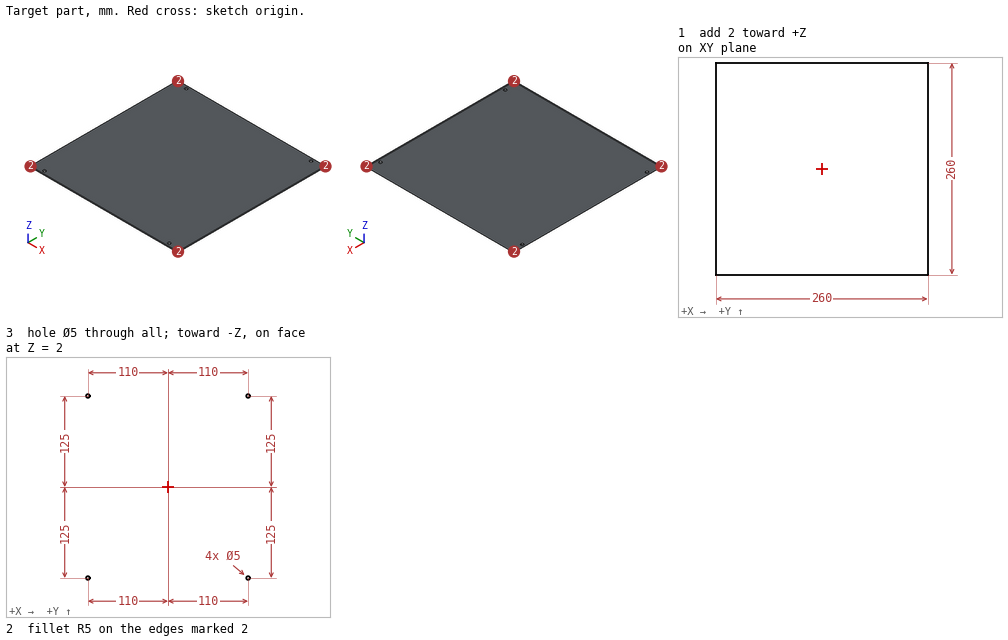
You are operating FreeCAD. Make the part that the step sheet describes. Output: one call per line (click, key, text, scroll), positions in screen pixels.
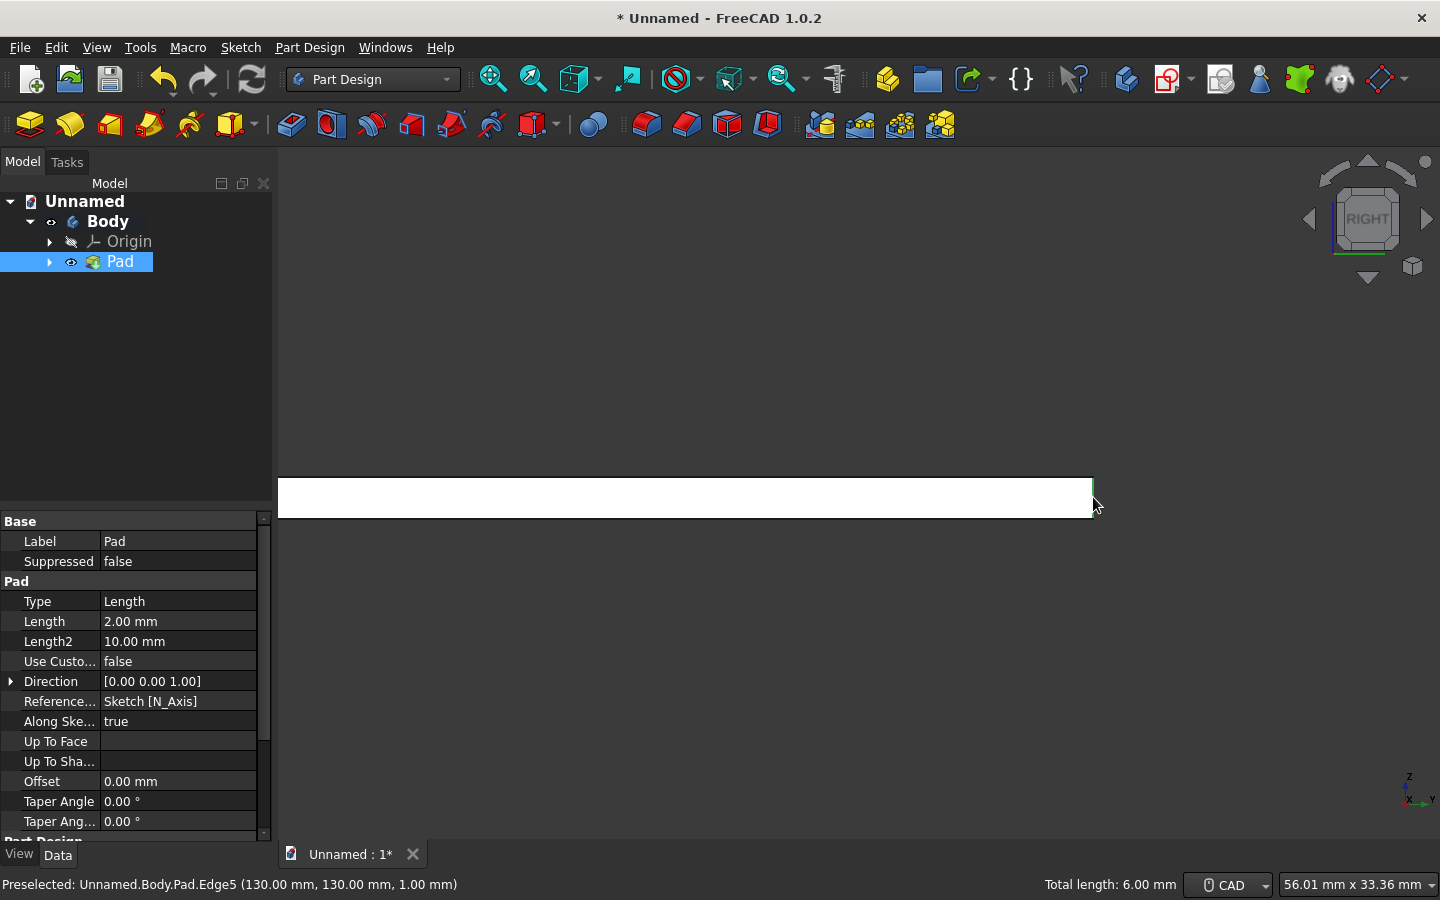
click(494, 80)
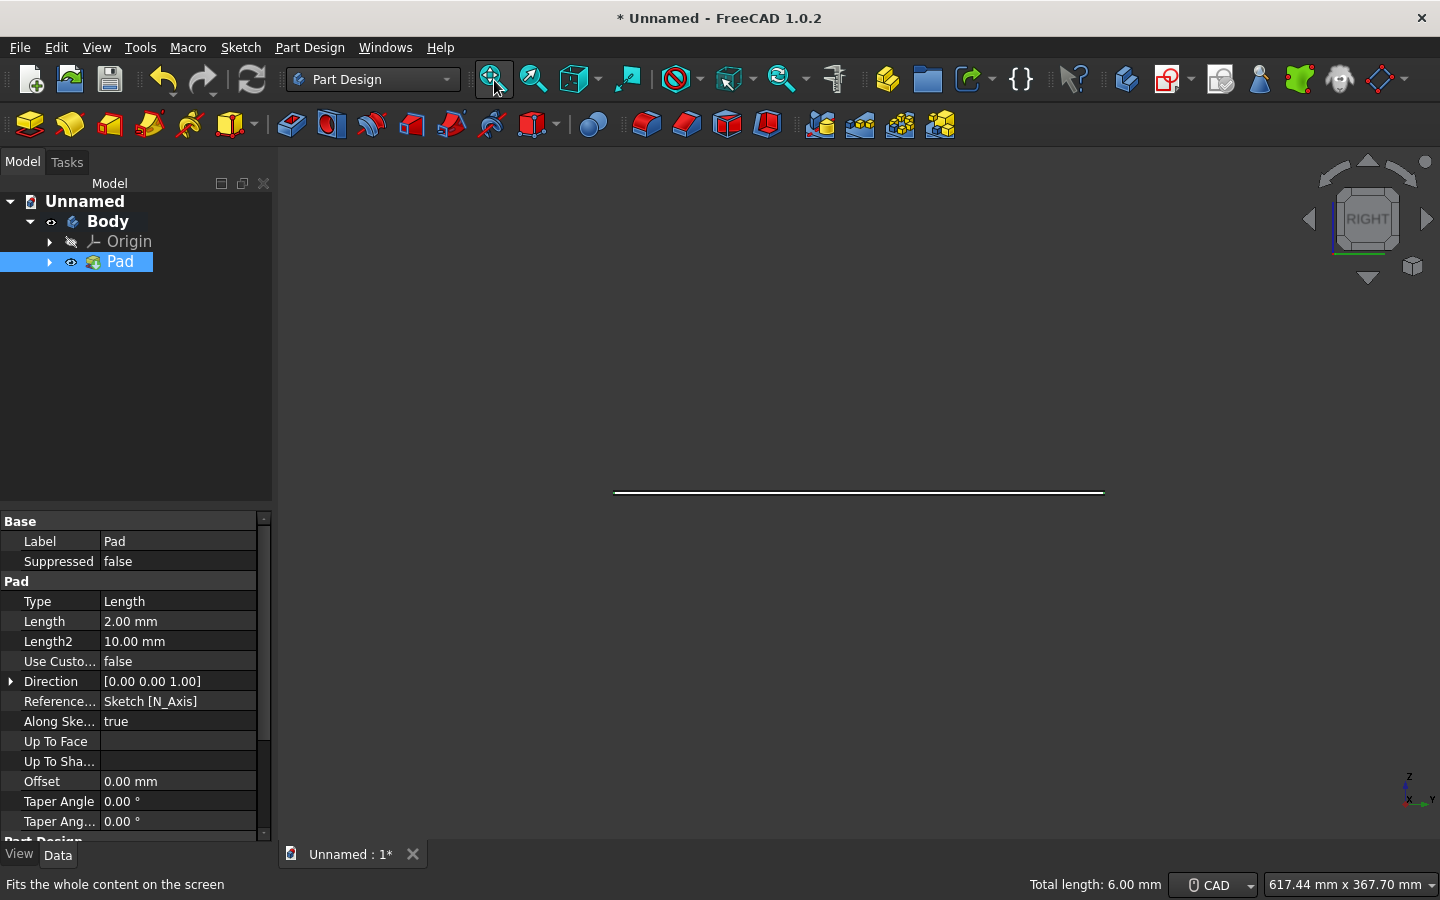
key(5)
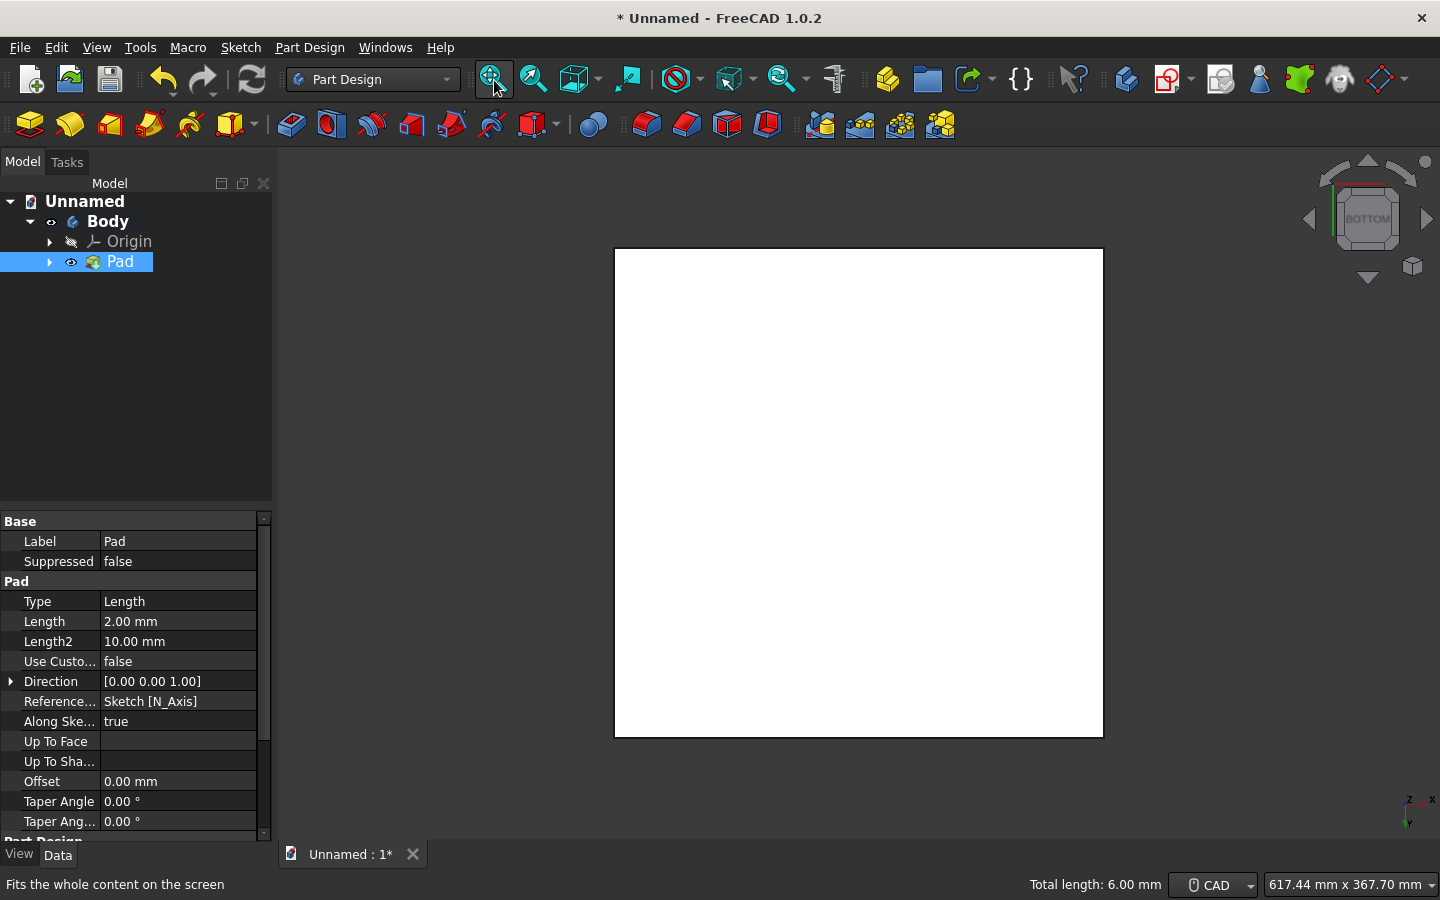
scroll(614, 737, up, 12)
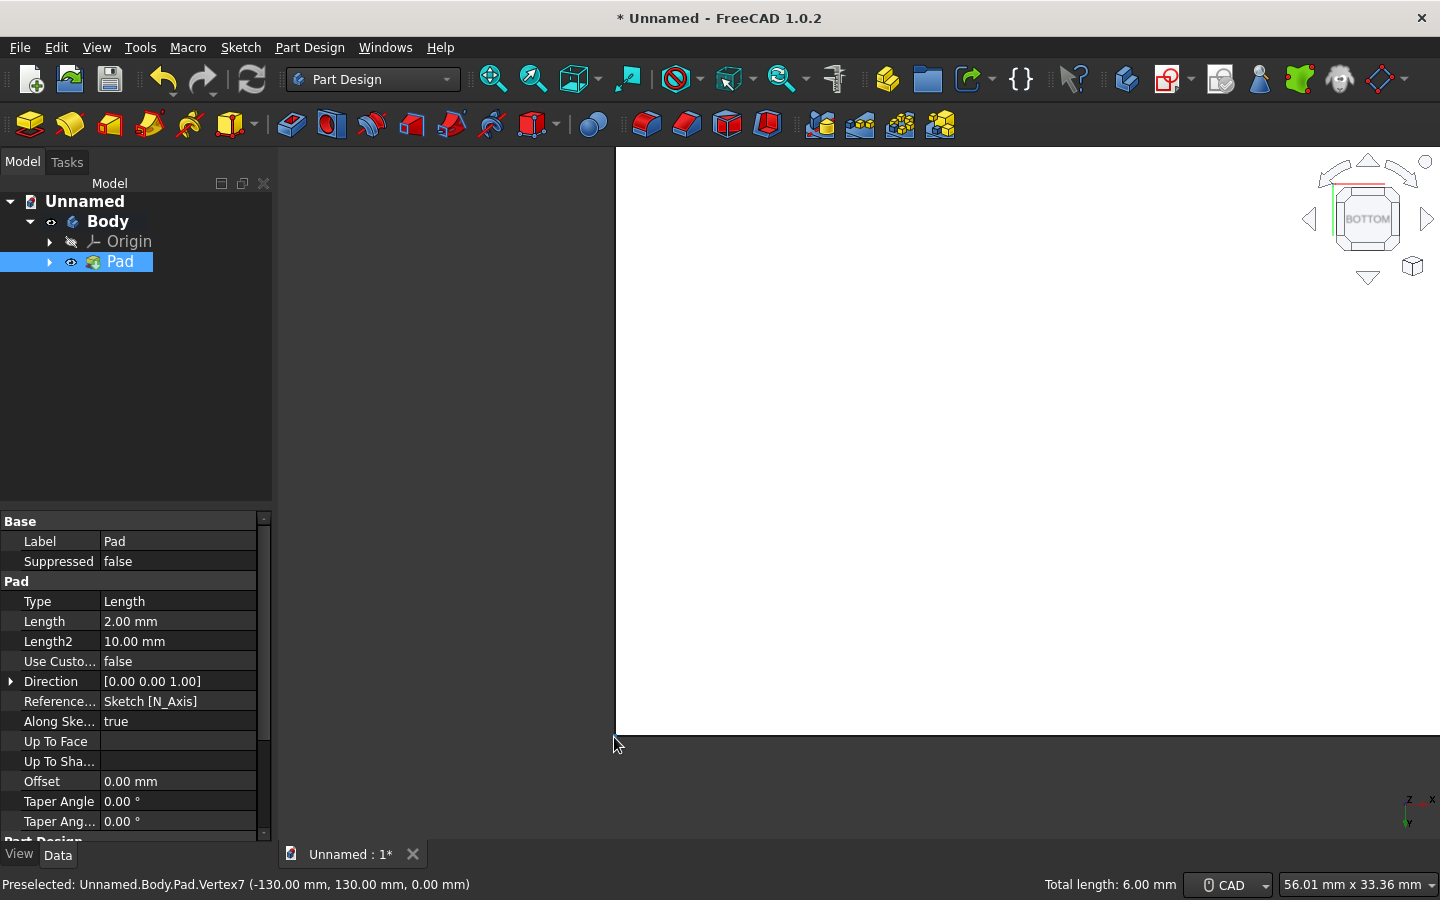
click(494, 80)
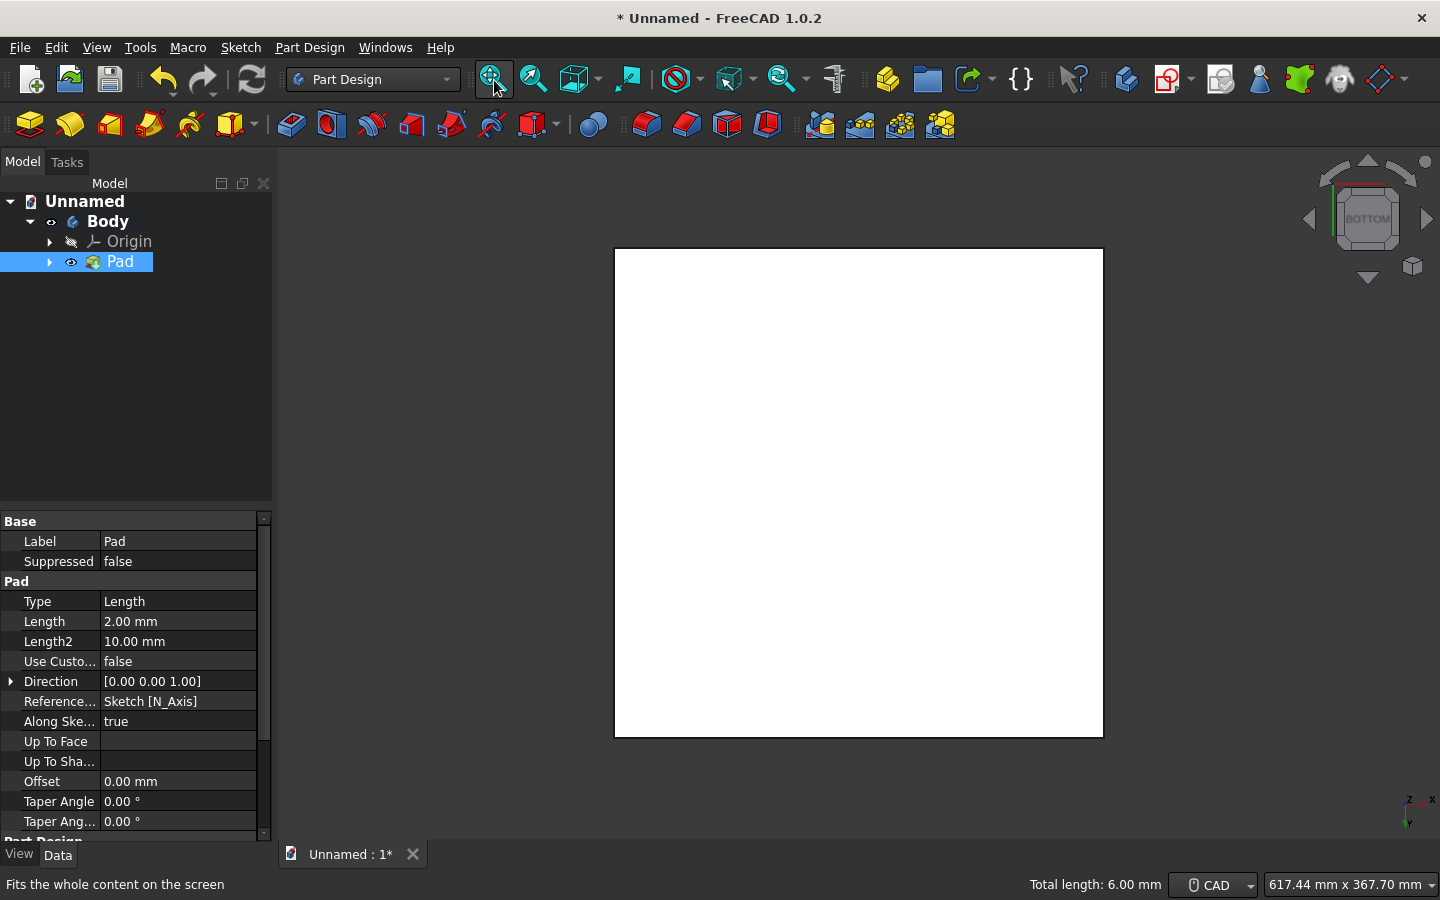
key(4)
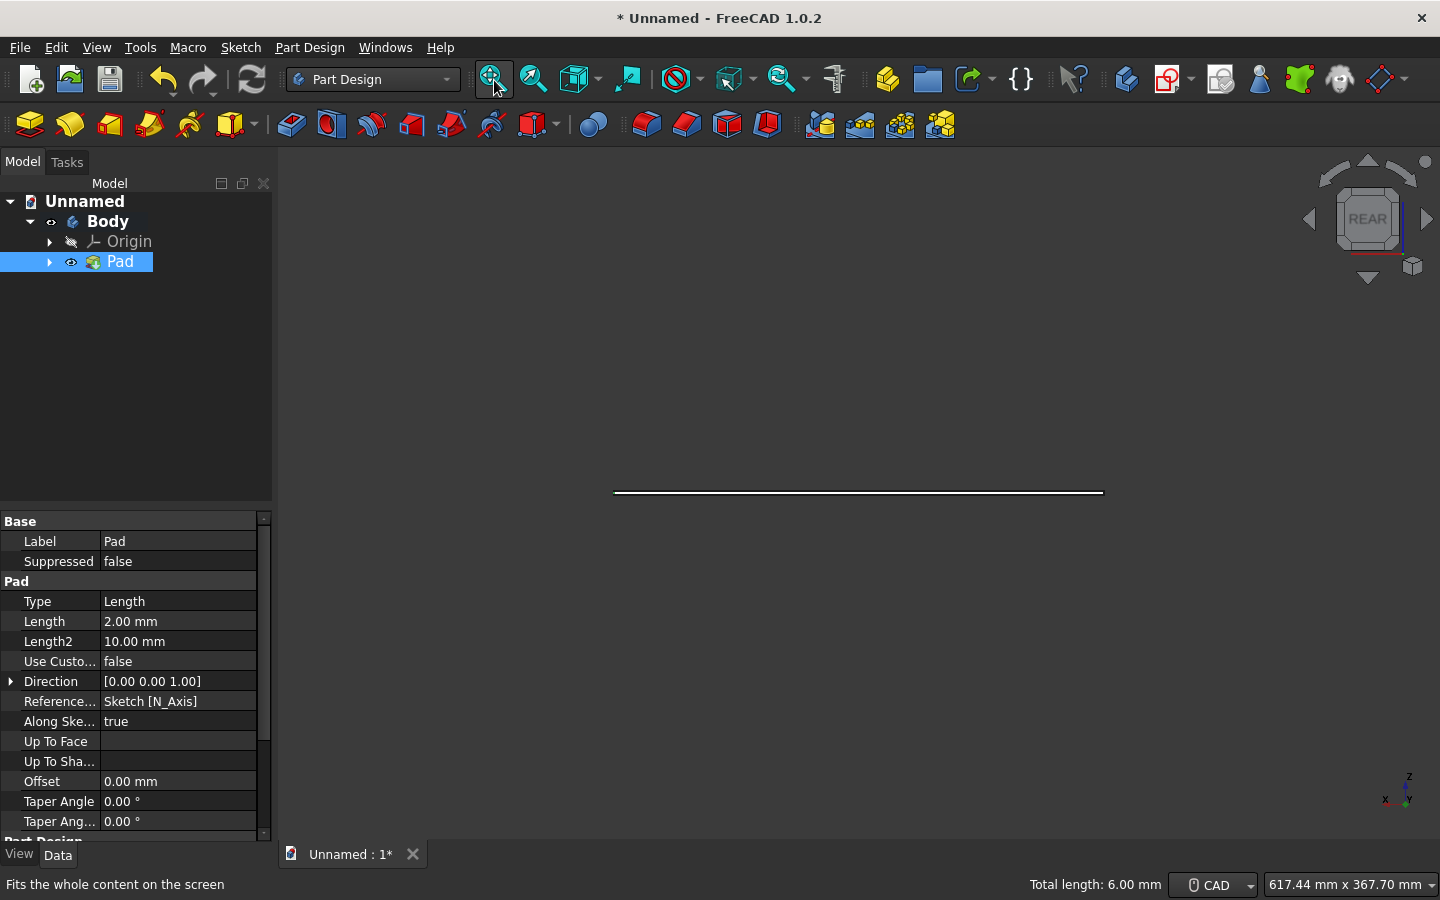
click(494, 80)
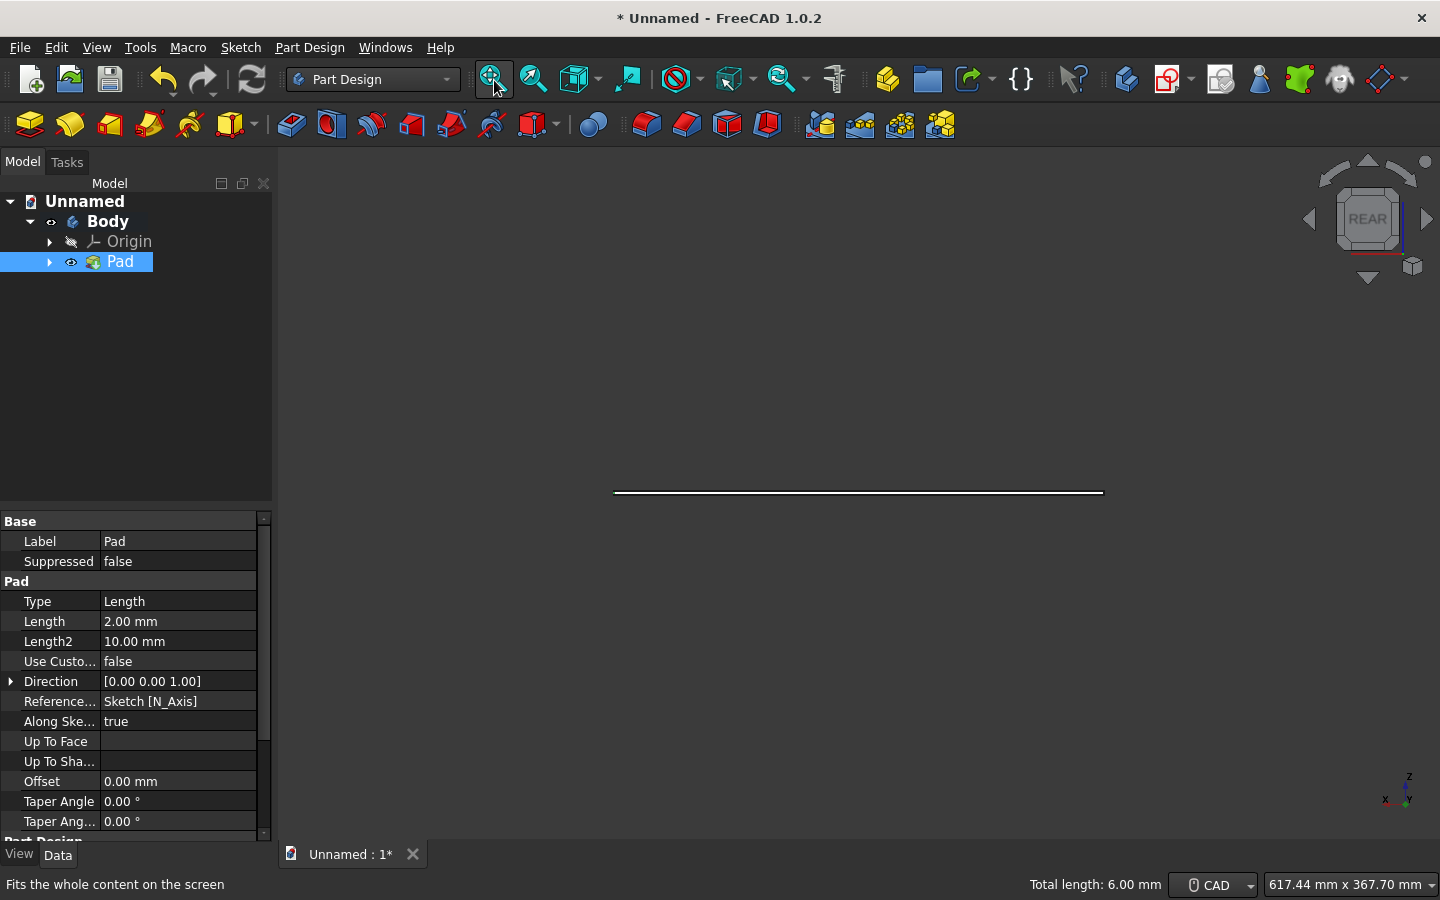
scroll(1104, 492, up, 12)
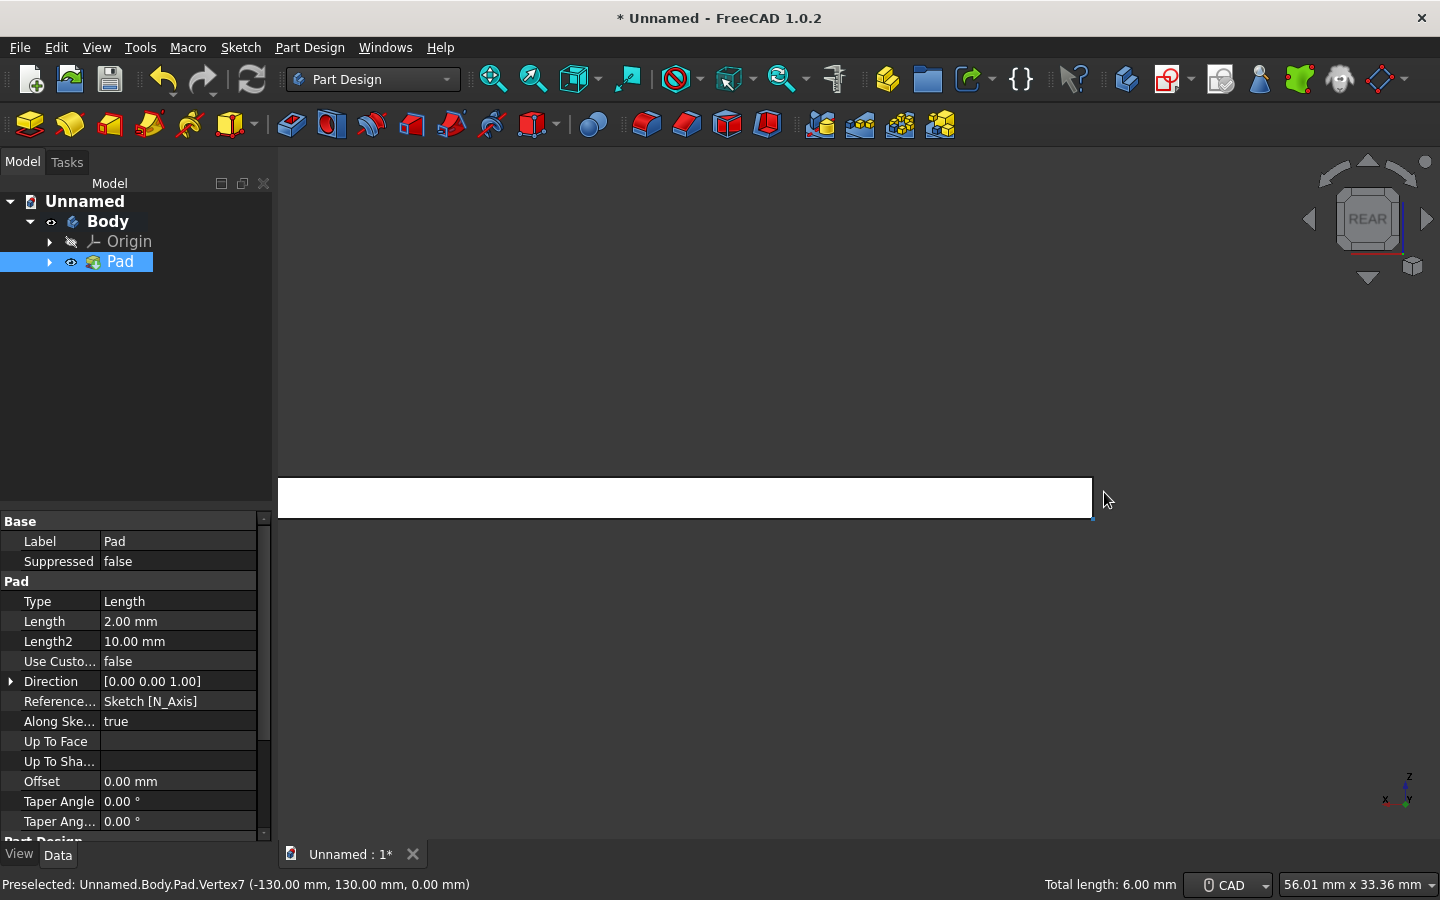
click(1093, 497, ctrl)